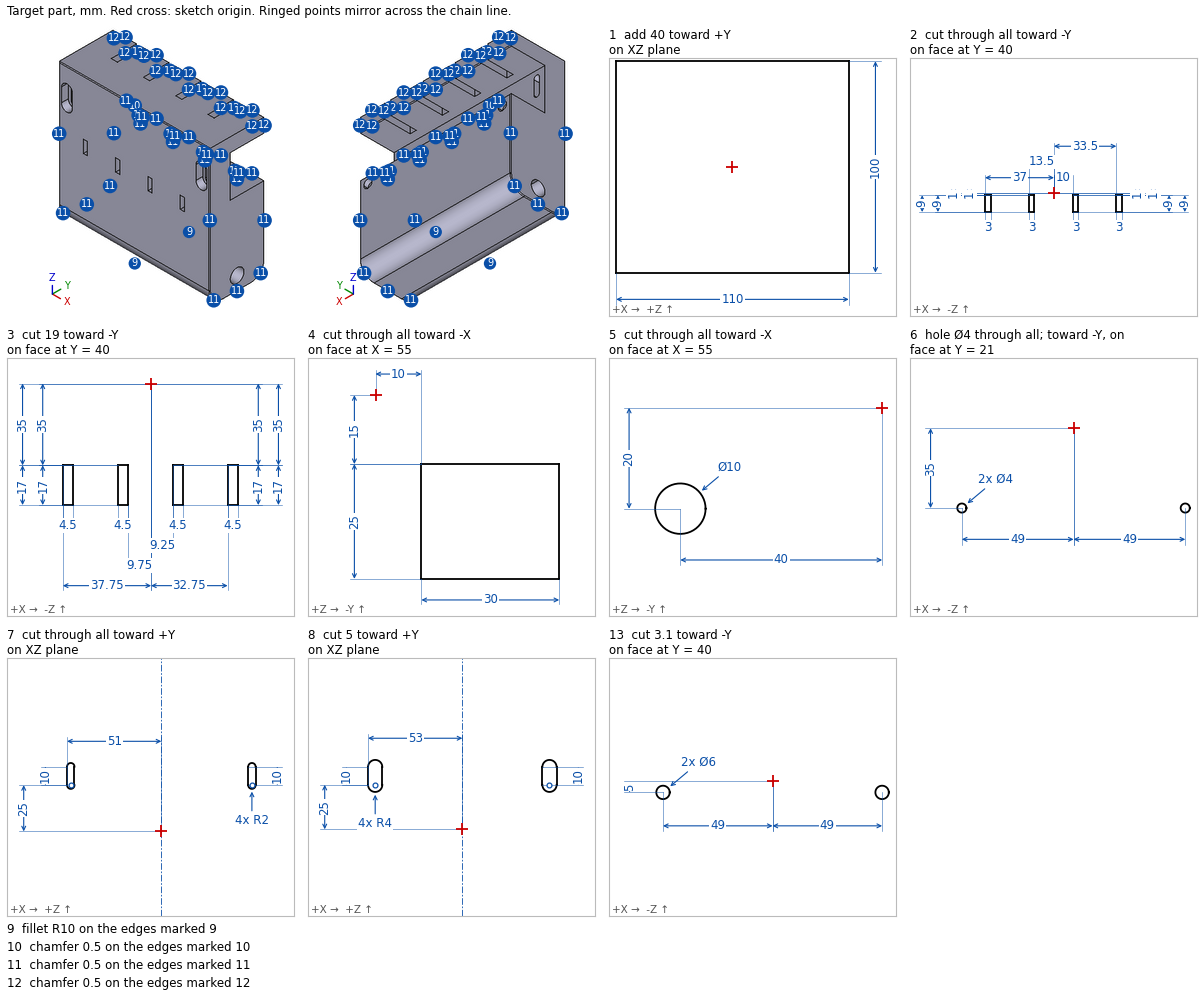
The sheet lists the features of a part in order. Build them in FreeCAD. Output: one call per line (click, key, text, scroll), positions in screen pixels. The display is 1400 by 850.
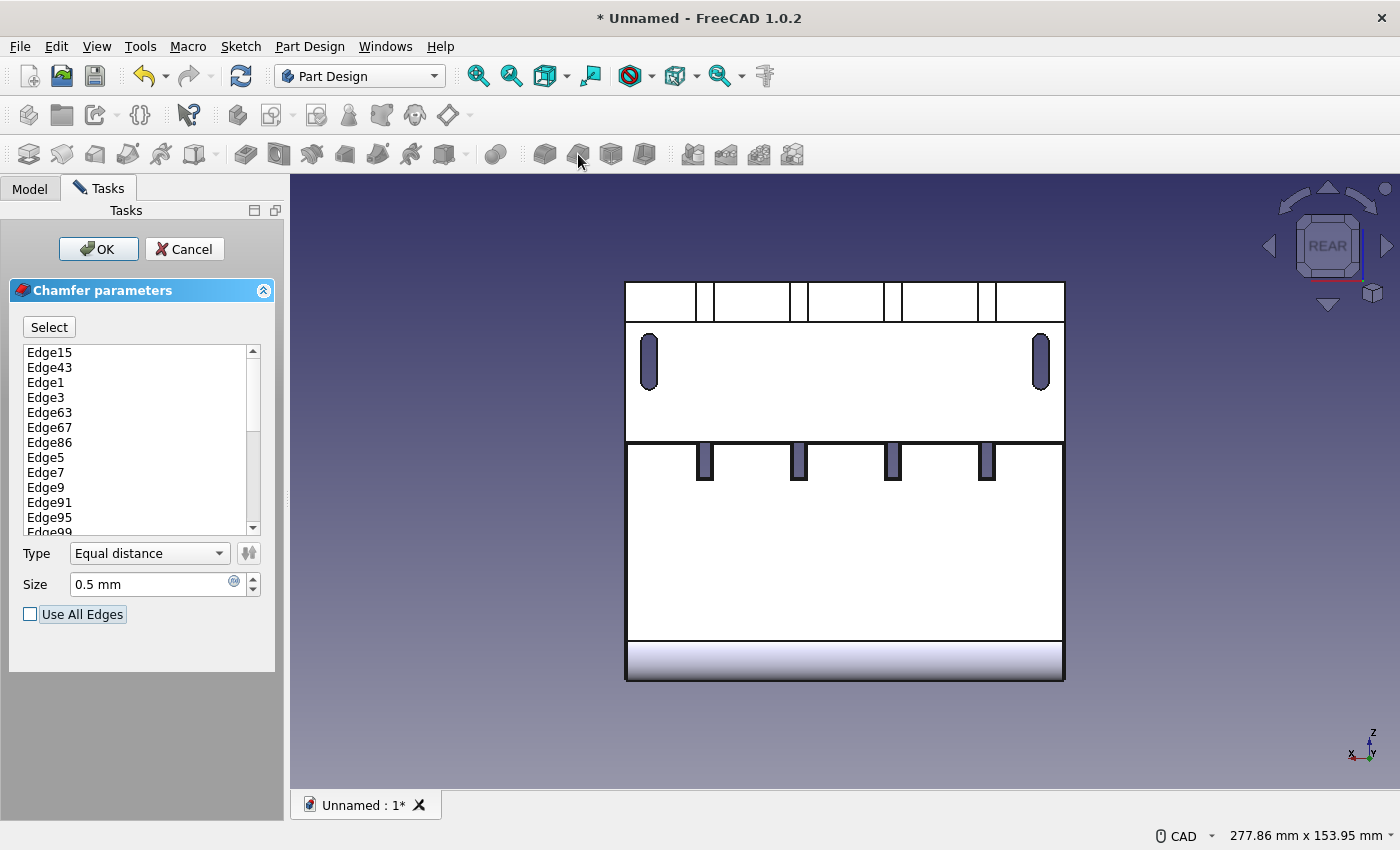
click(99, 249)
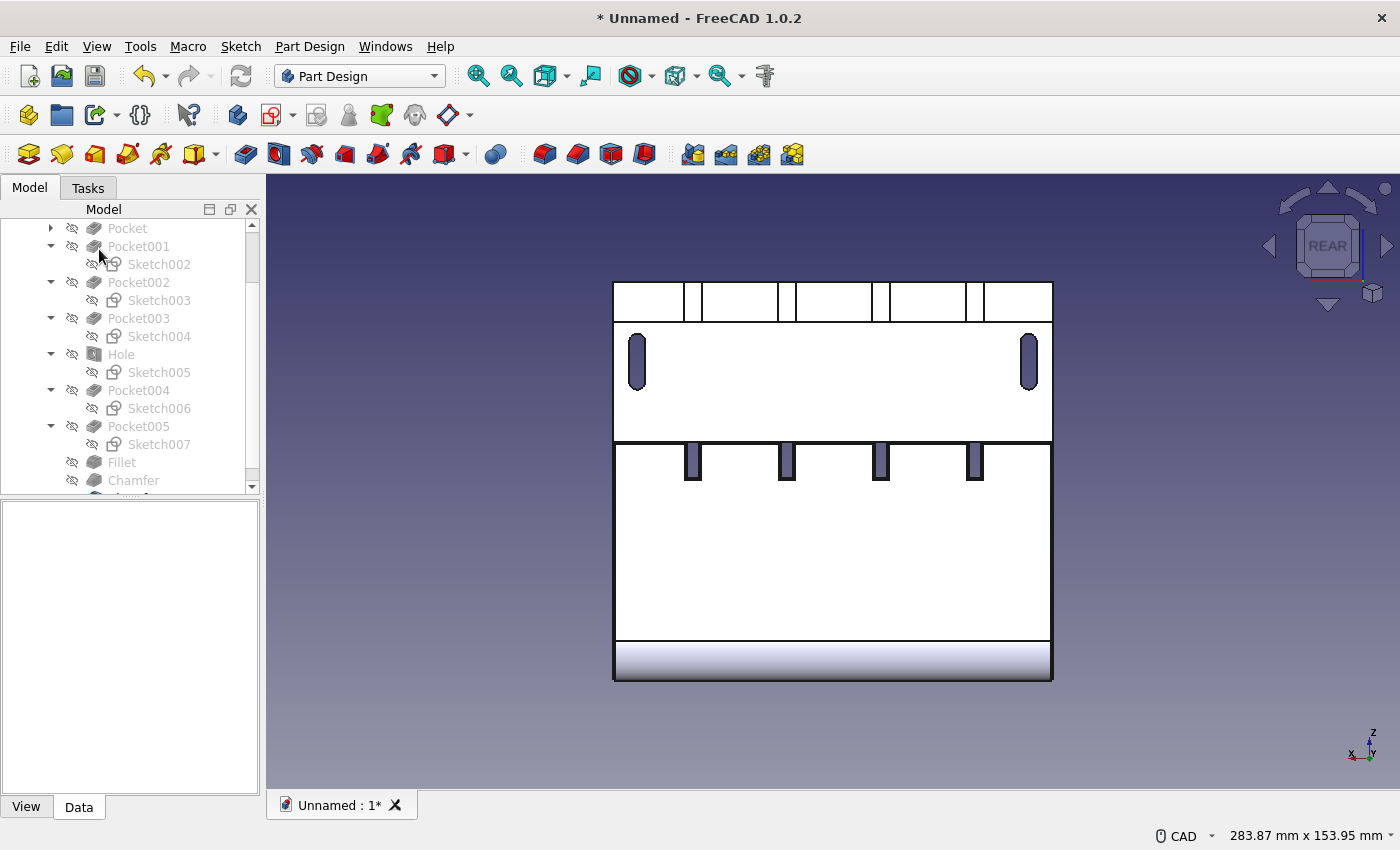
click(729, 301)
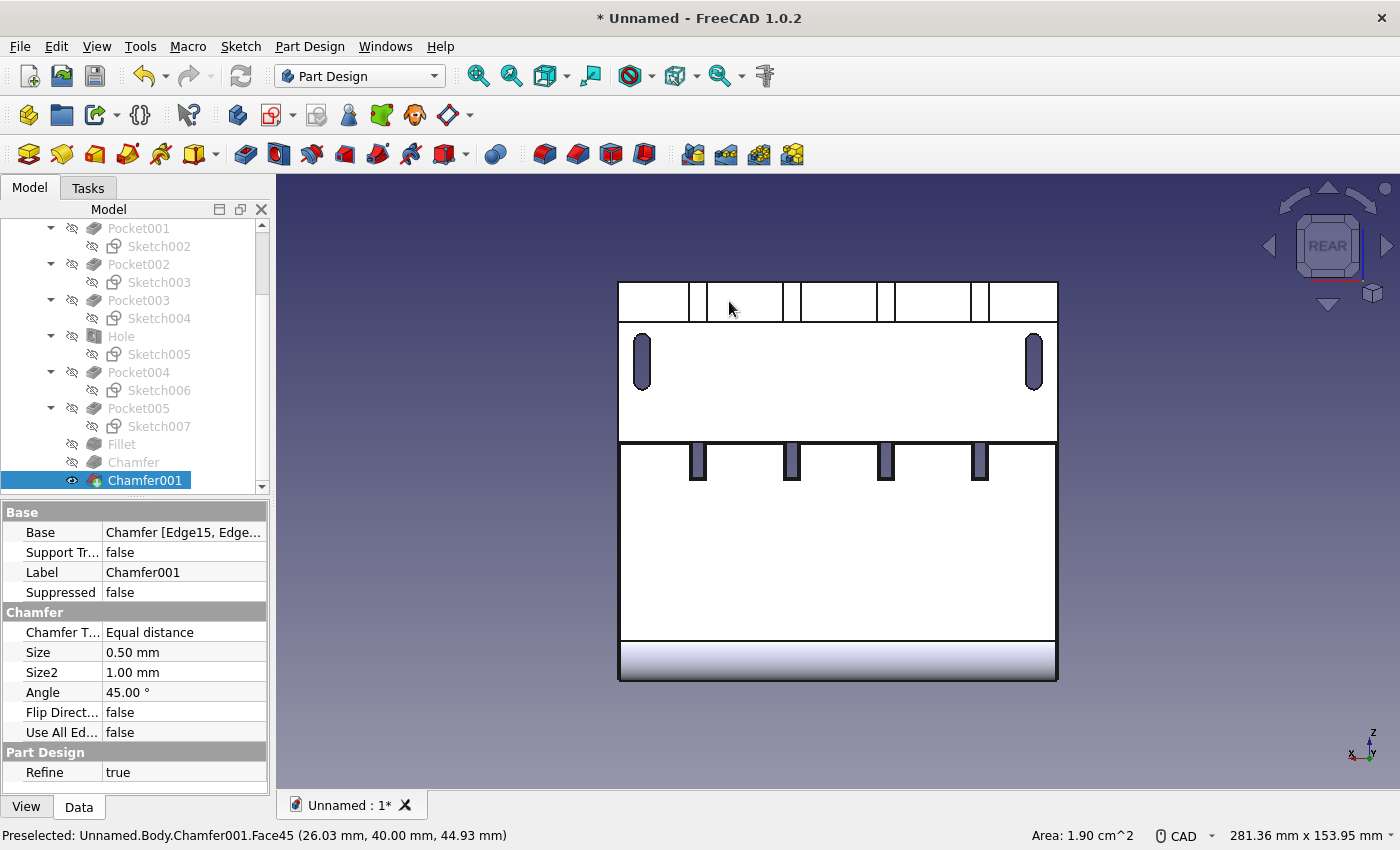
click(828, 301, ctrl)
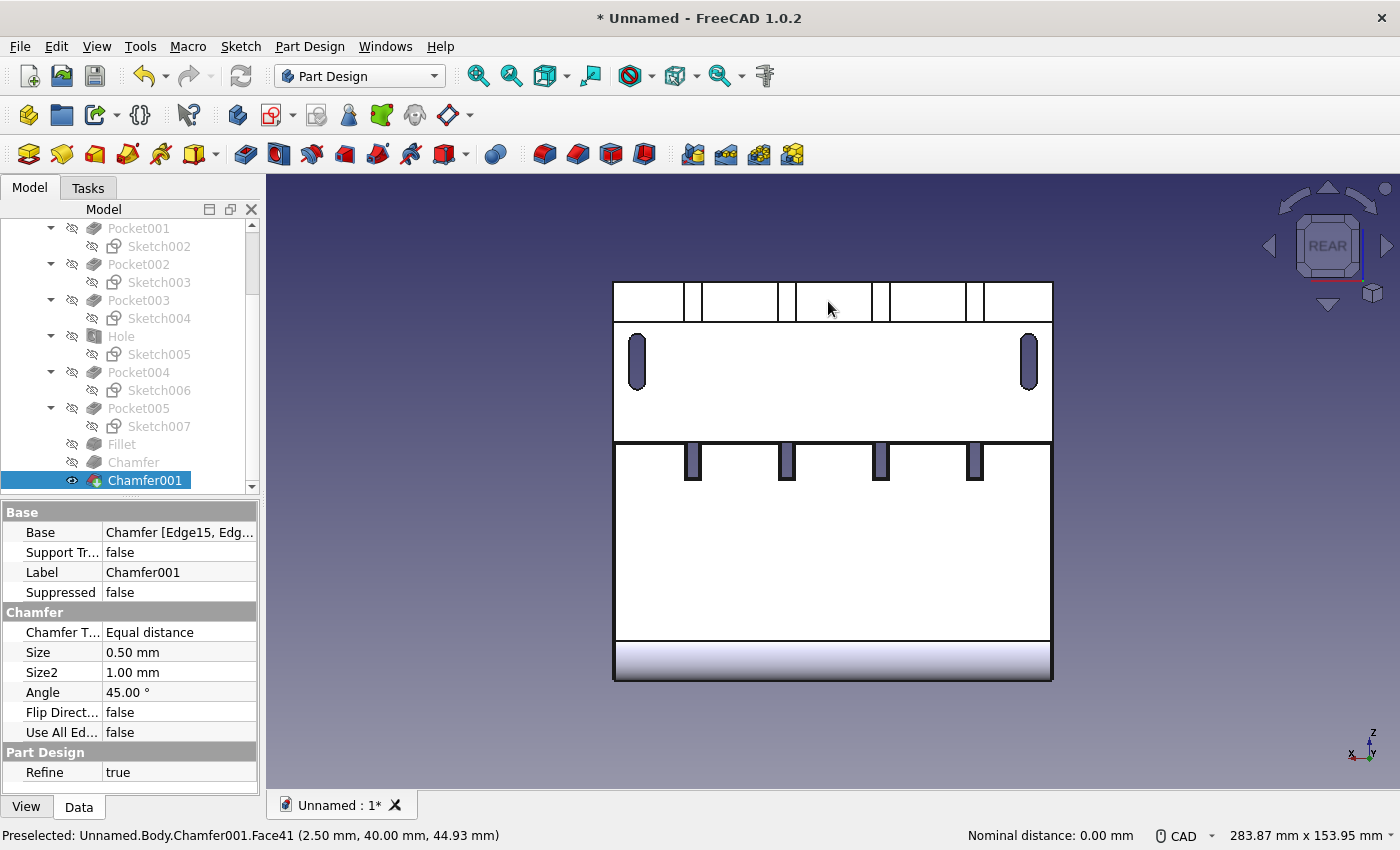
click(917, 301, ctrl)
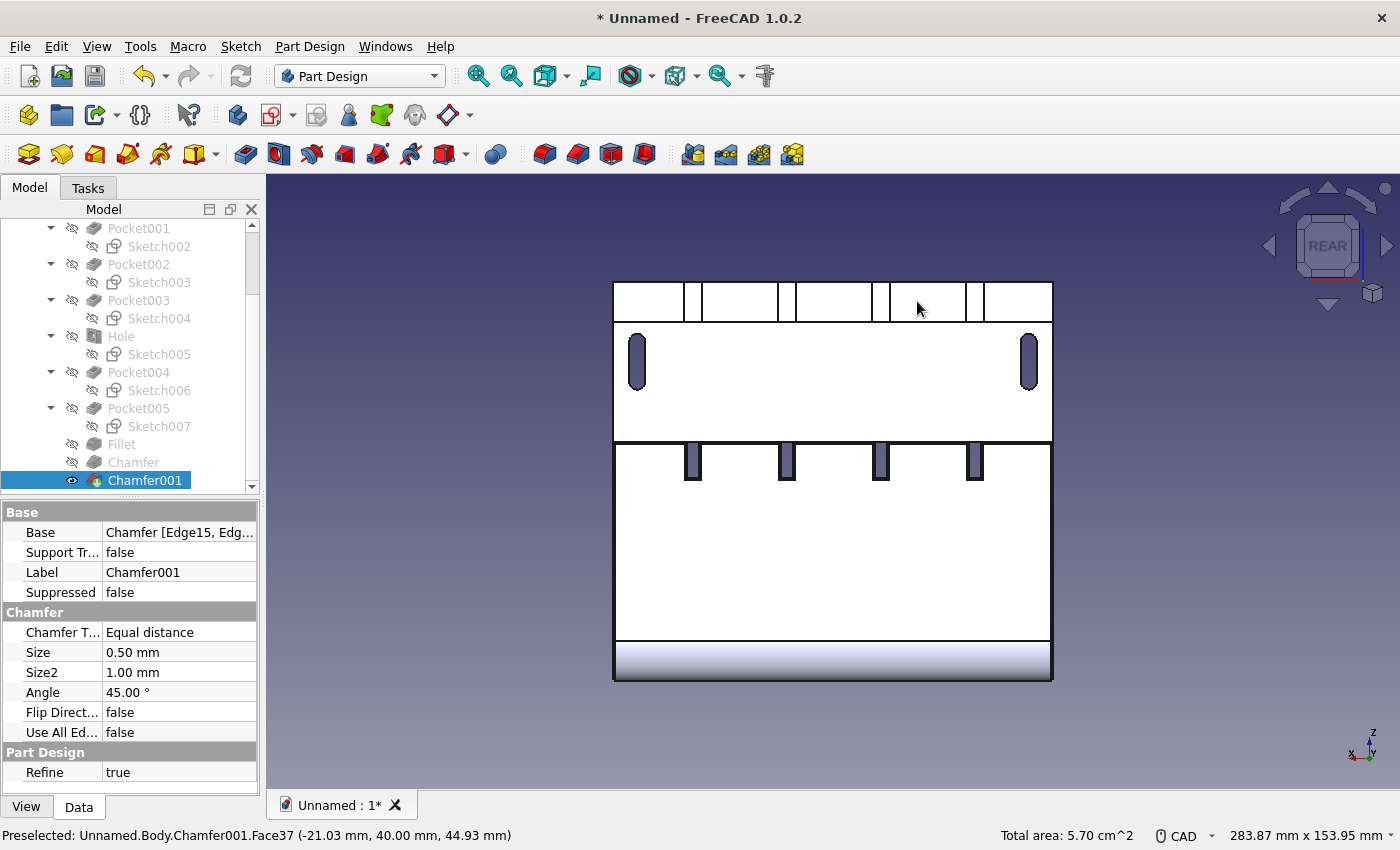
click(639, 301, ctrl)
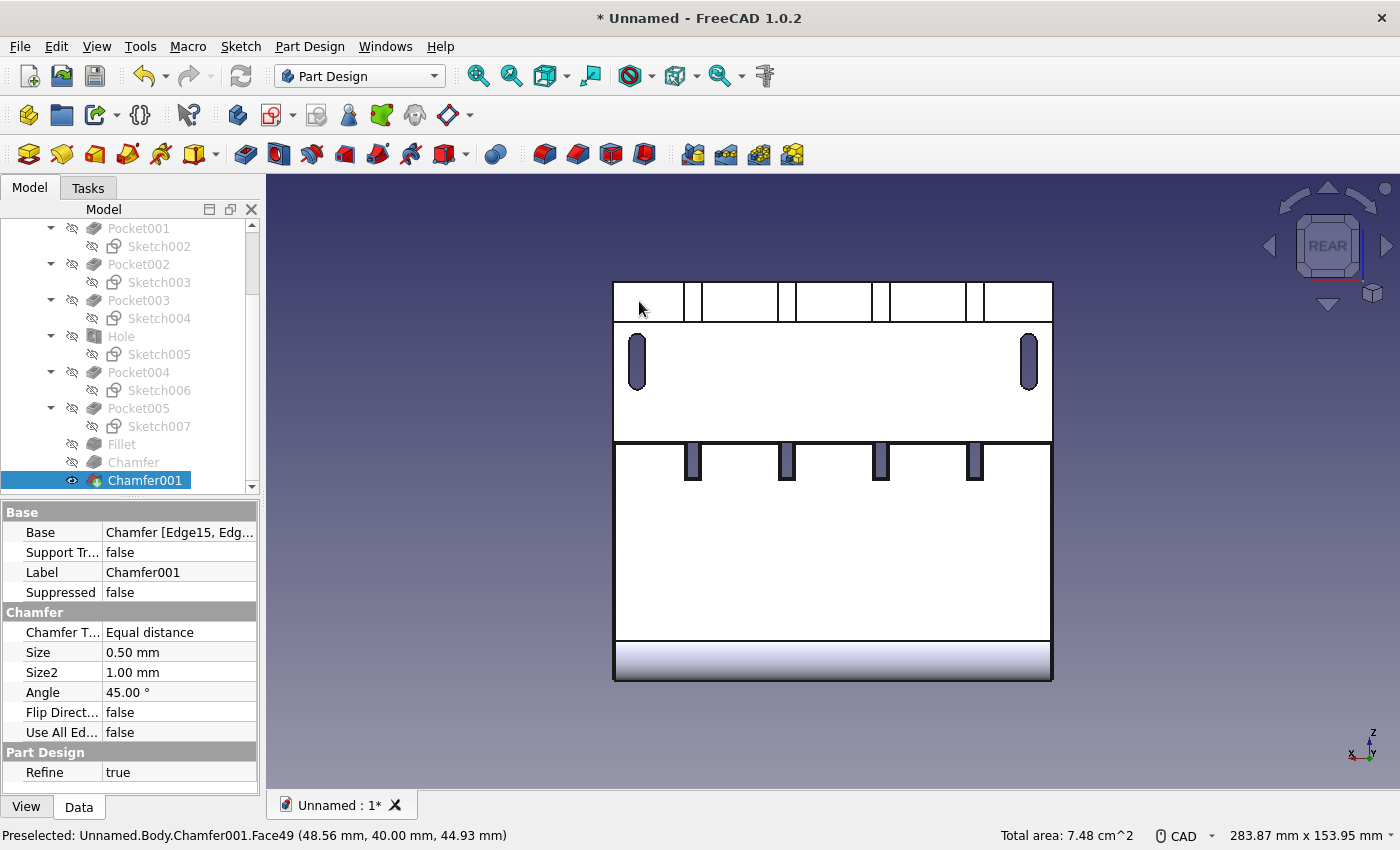
click(1008, 301, ctrl)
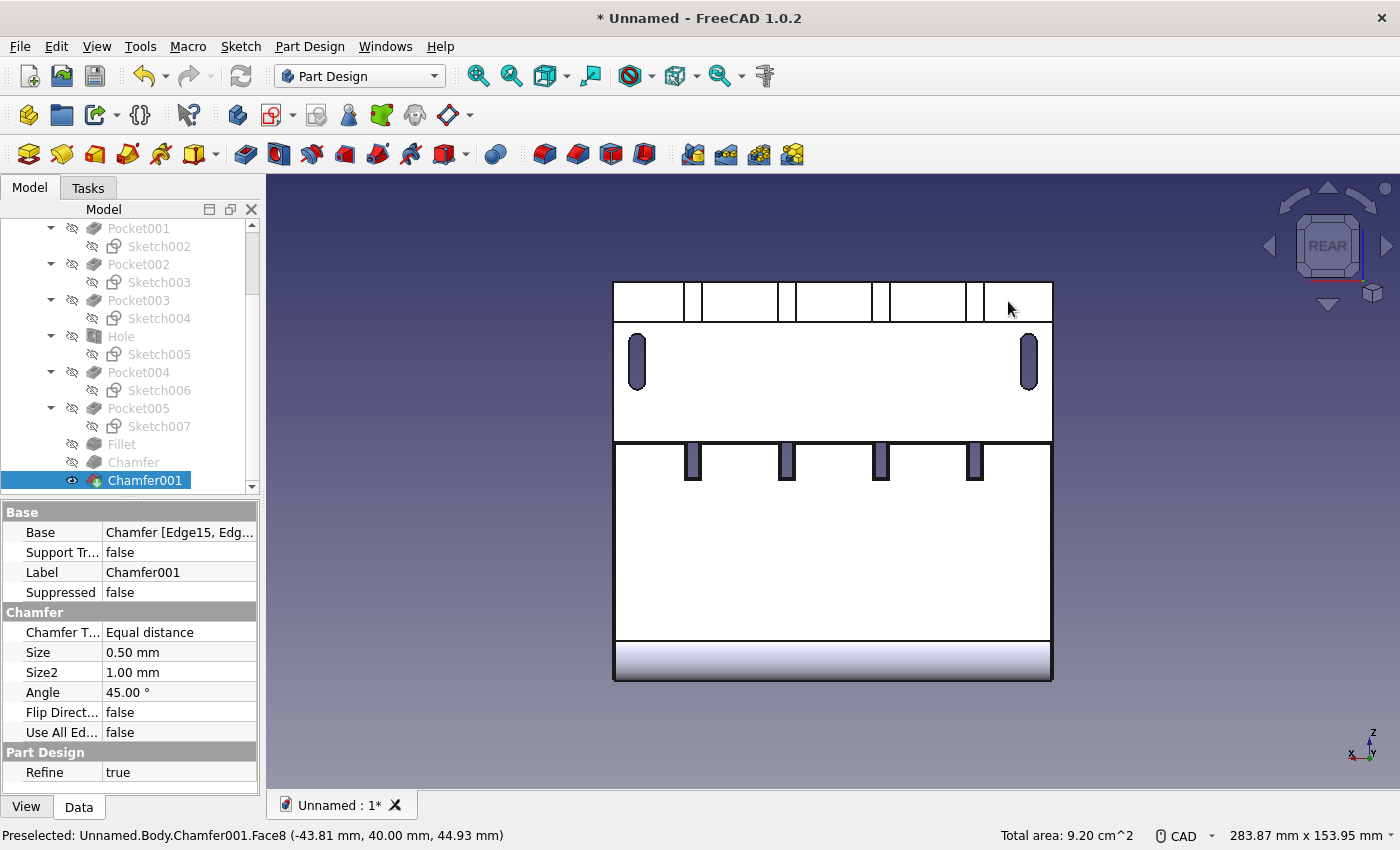
click(578, 154)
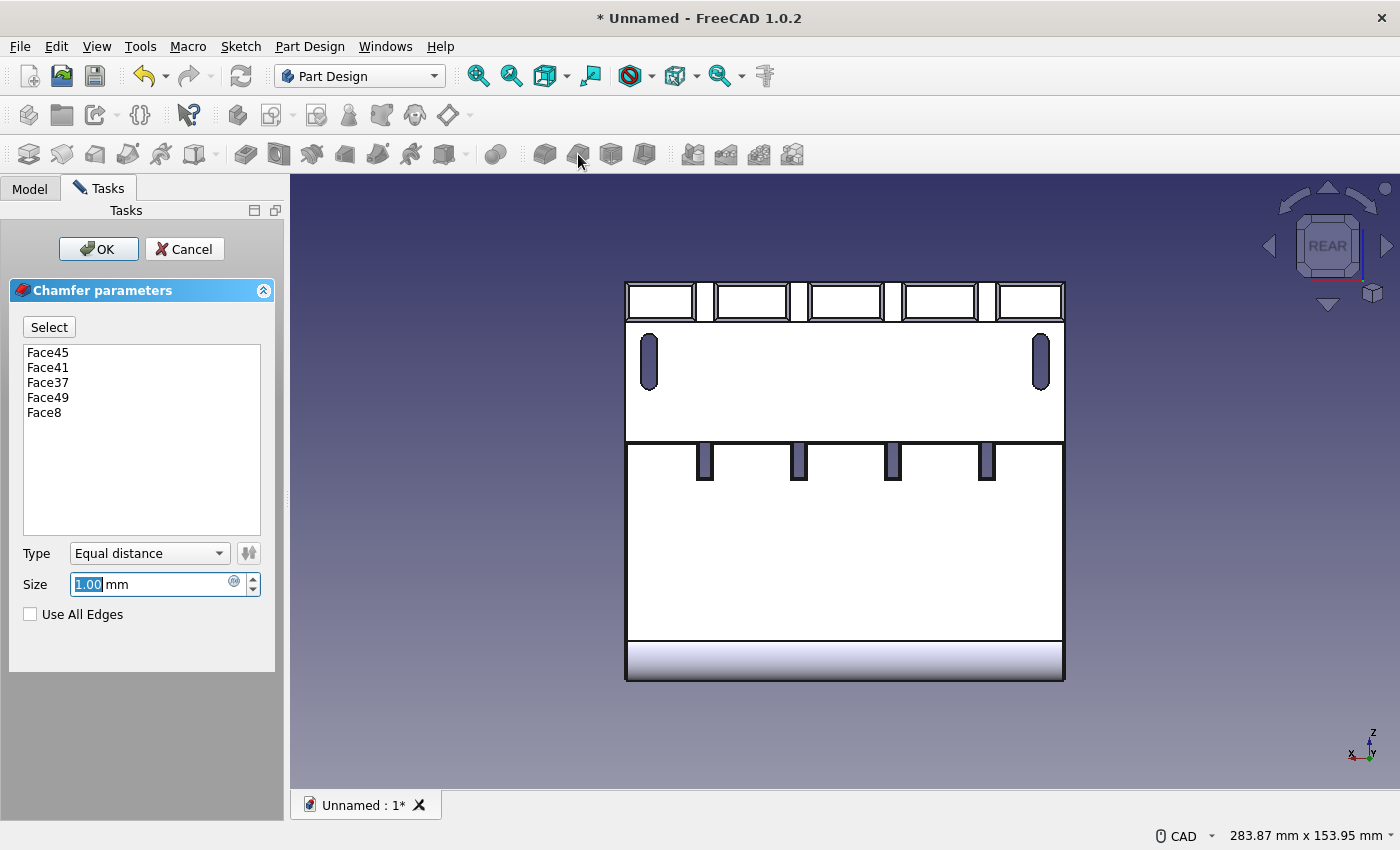
text(0.5)
key(Tab)